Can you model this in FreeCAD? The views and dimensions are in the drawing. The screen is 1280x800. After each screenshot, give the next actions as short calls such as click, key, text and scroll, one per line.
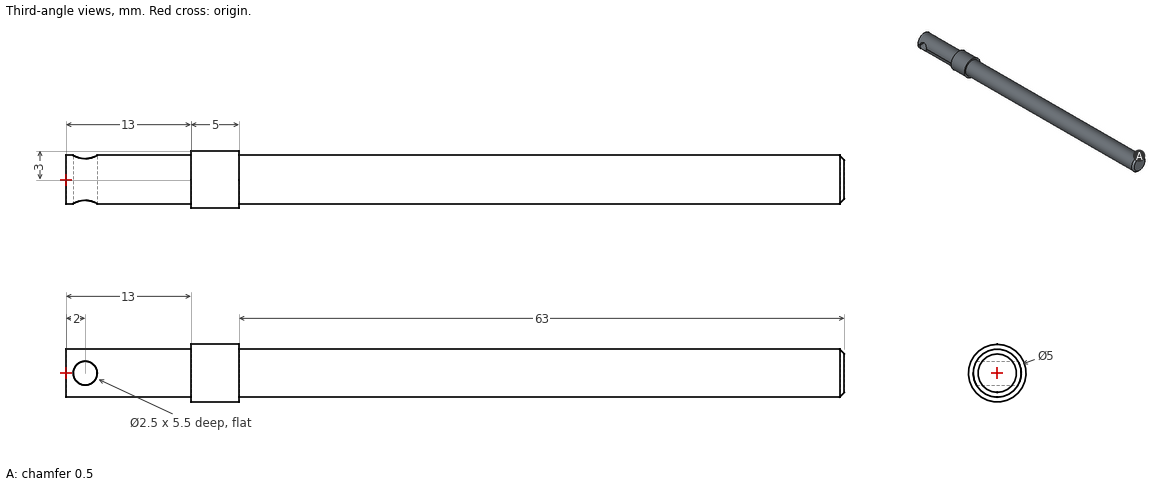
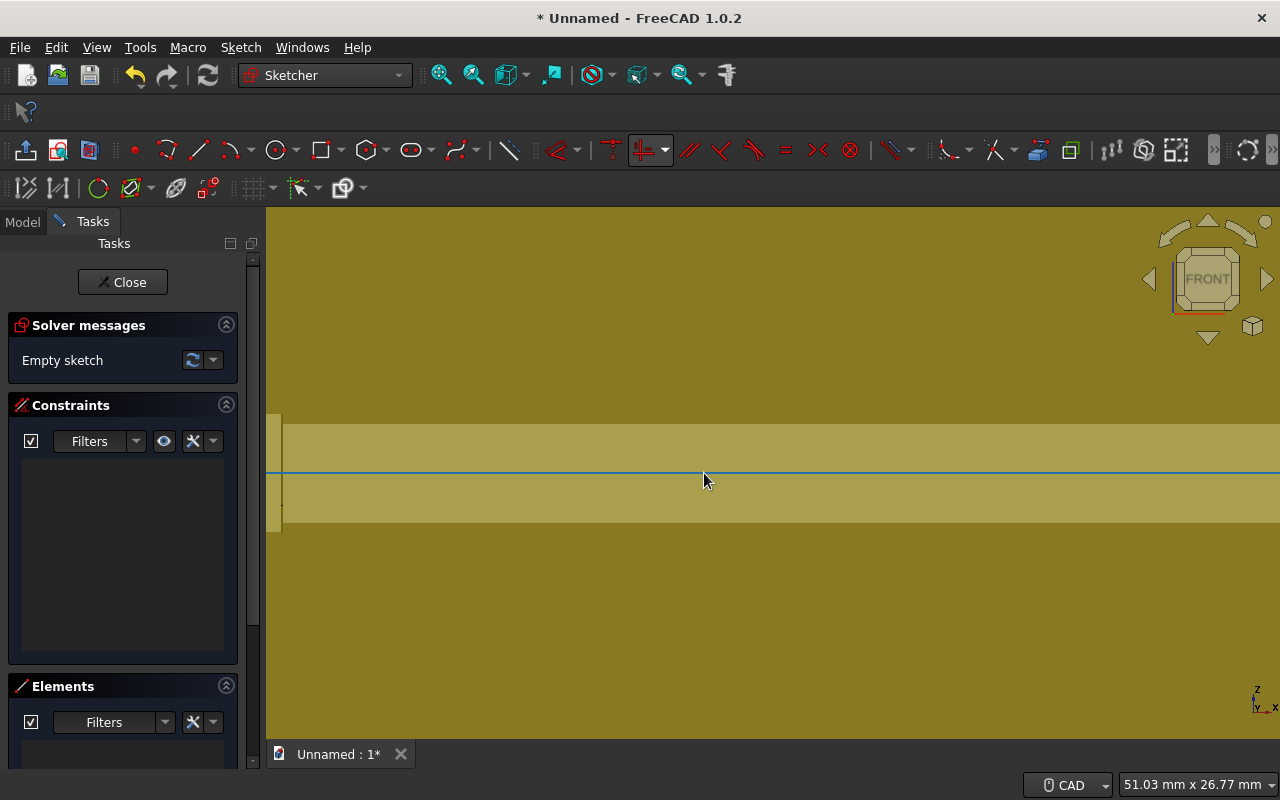
scroll(704, 473, down, 5)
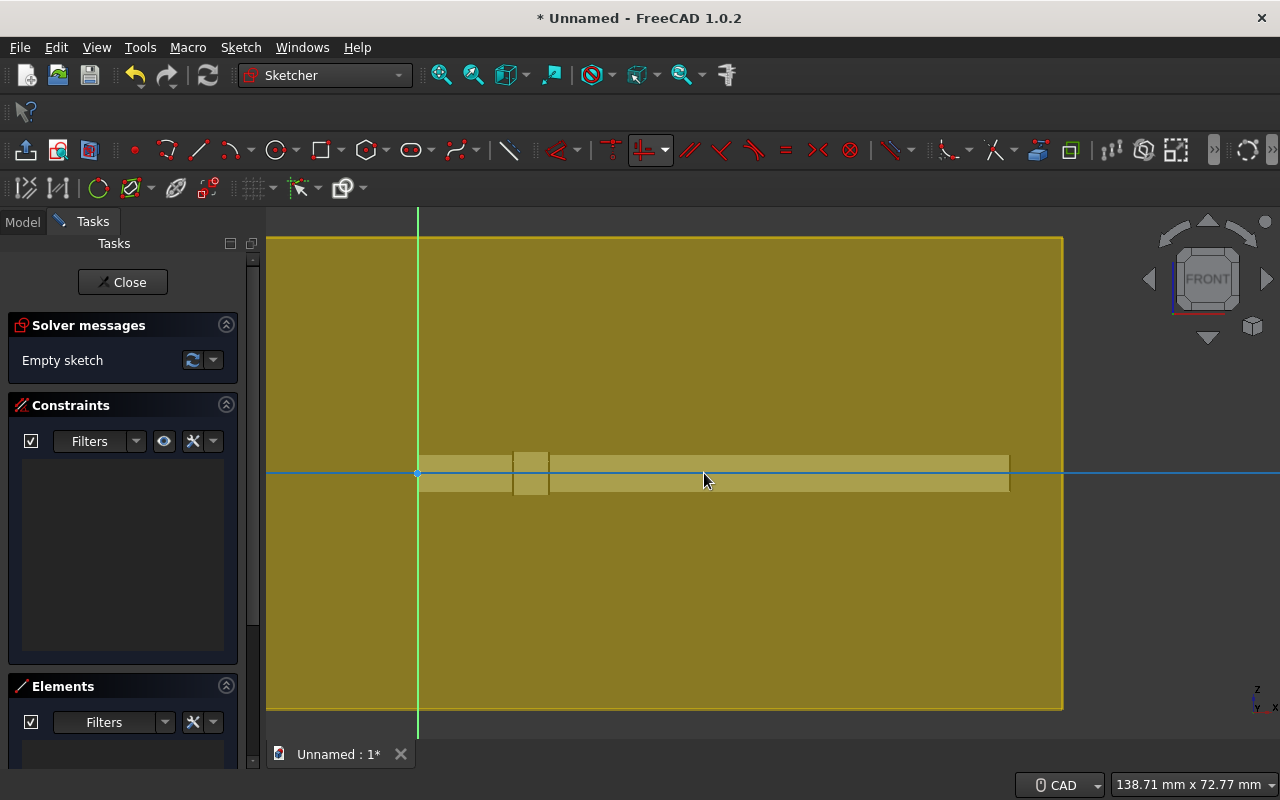
scroll(415, 473, up, 15)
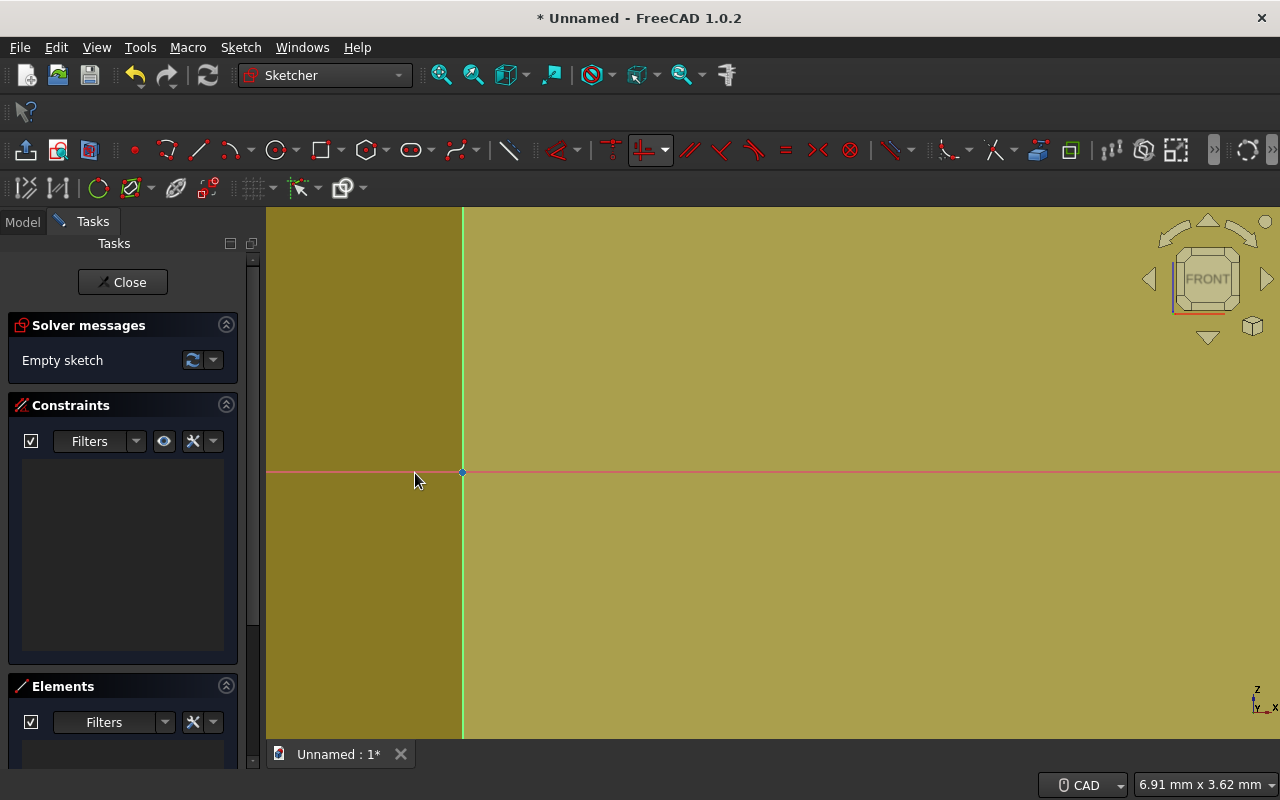
click(276, 150)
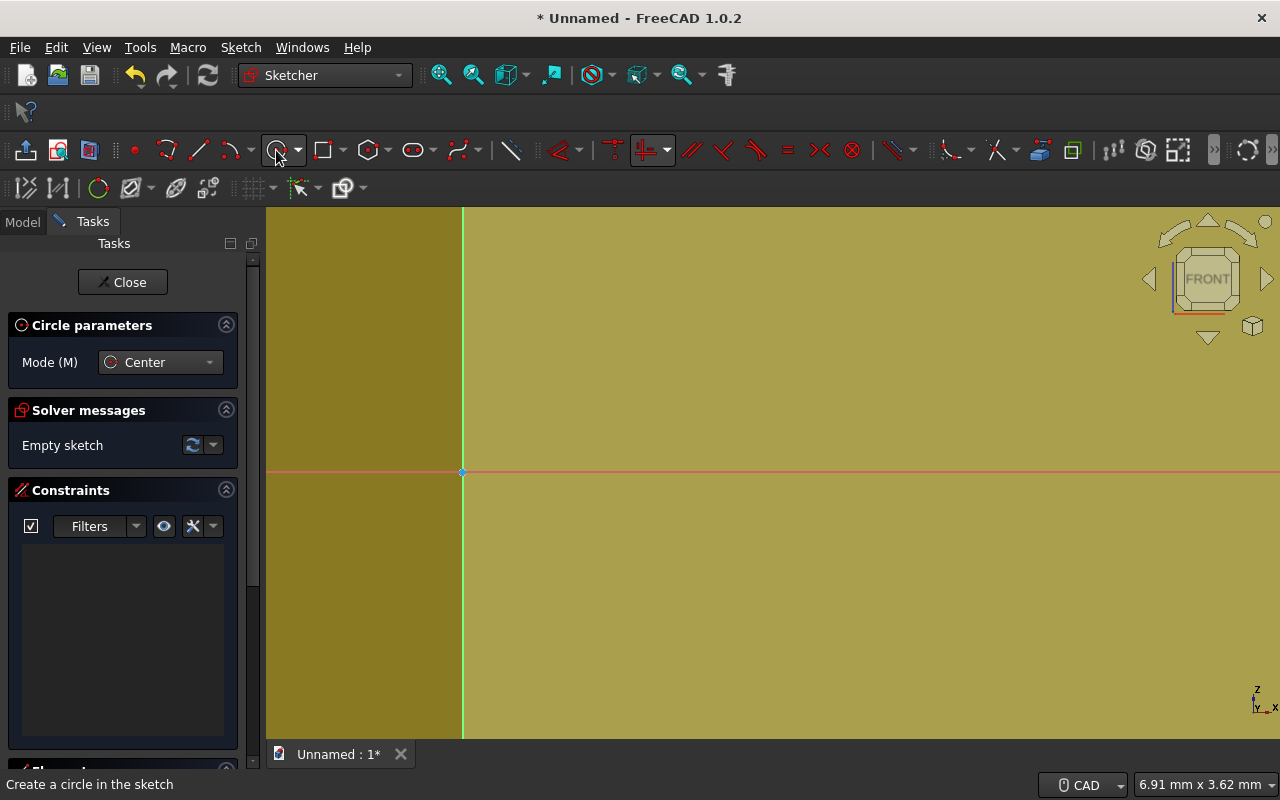
click(757, 472)
move(886, 342)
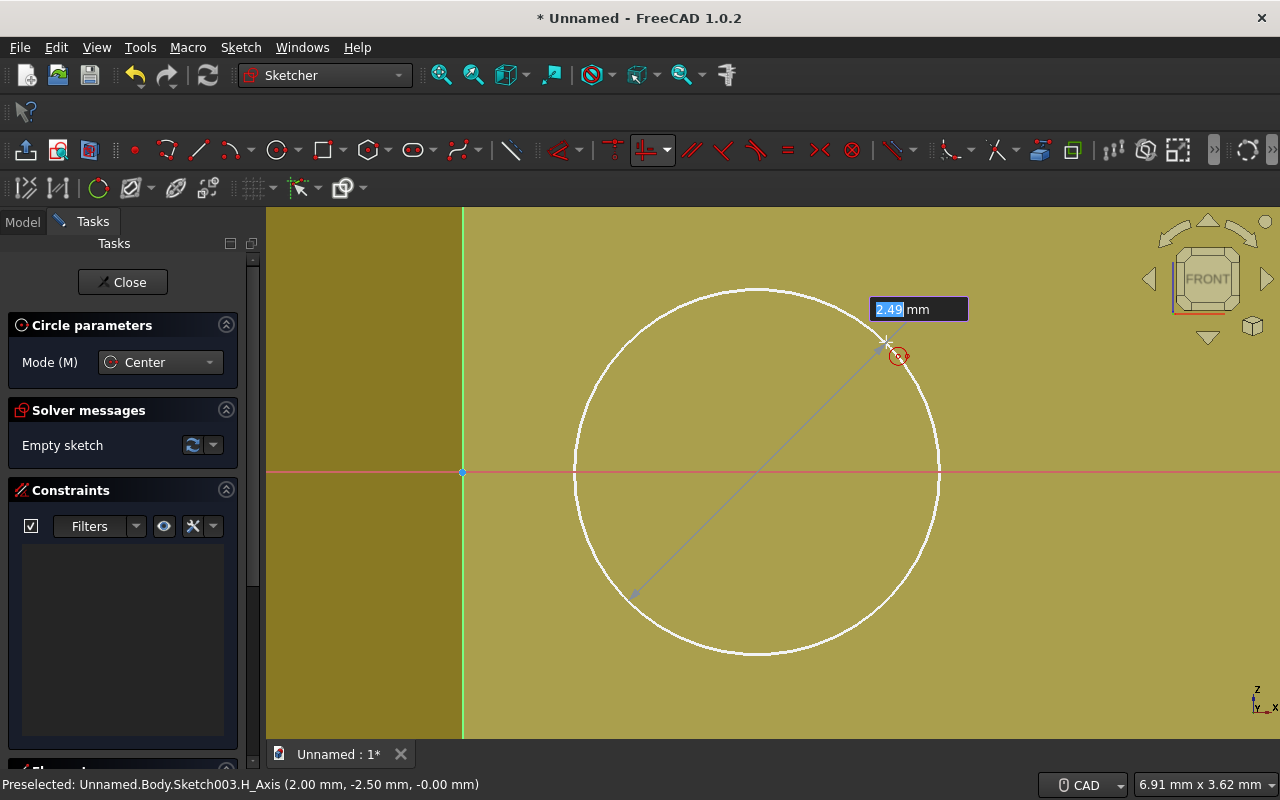
text(2.5)
key(Return)
key(Escape)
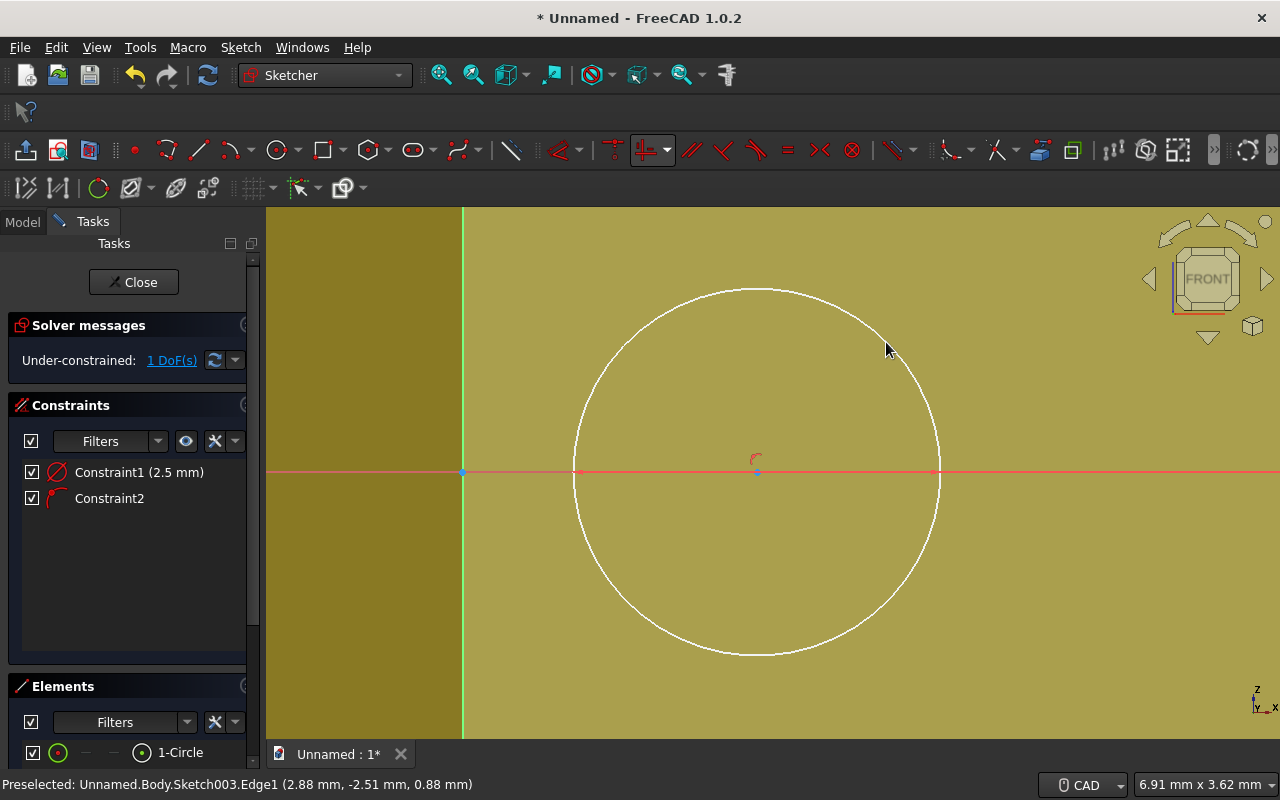
click(558, 150)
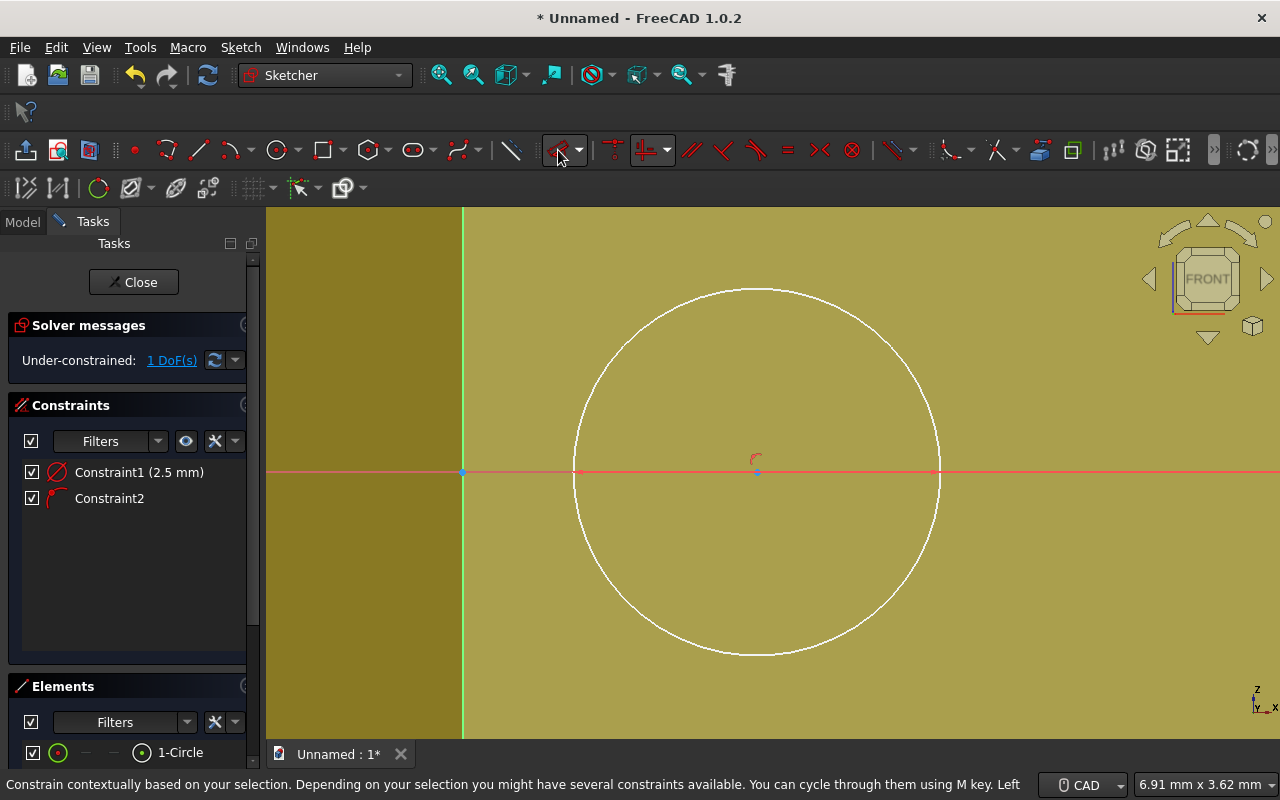
click(757, 472)
click(610, 506)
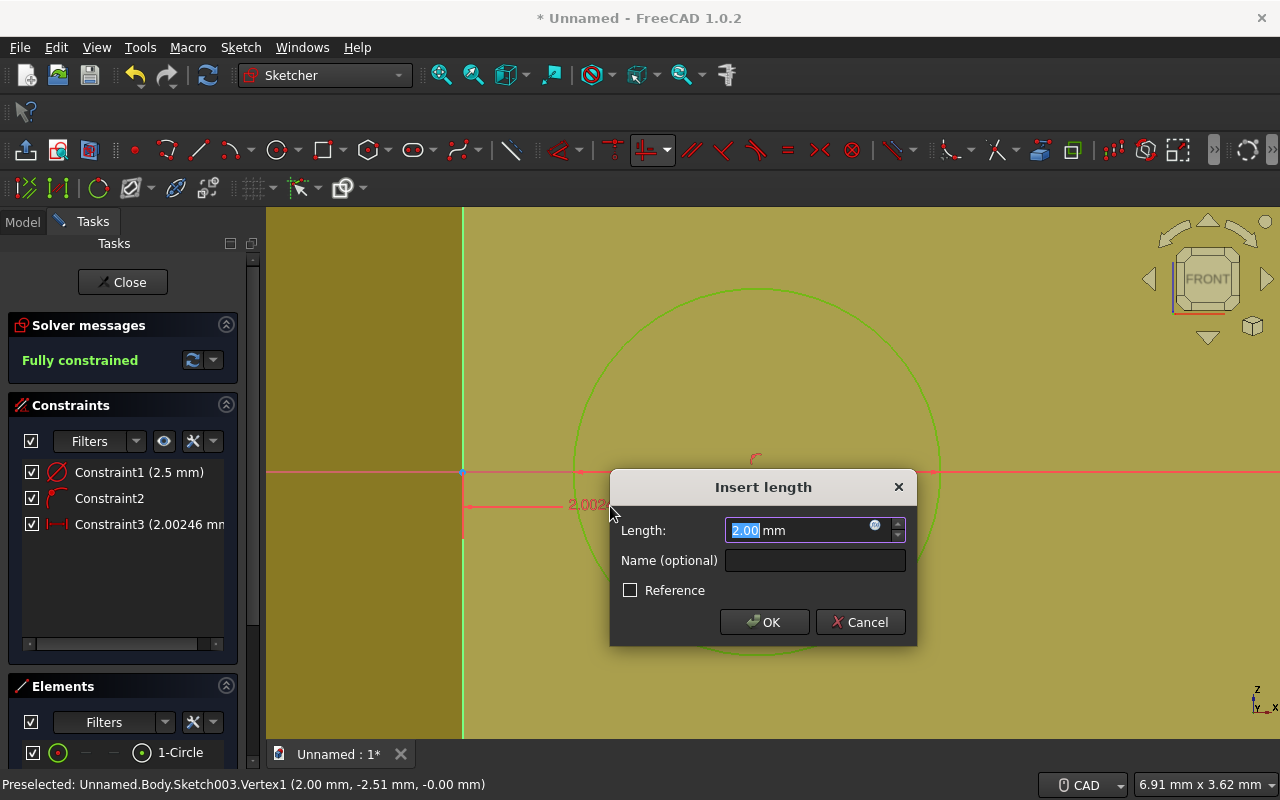
text(2)
key(Return)
key(Escape)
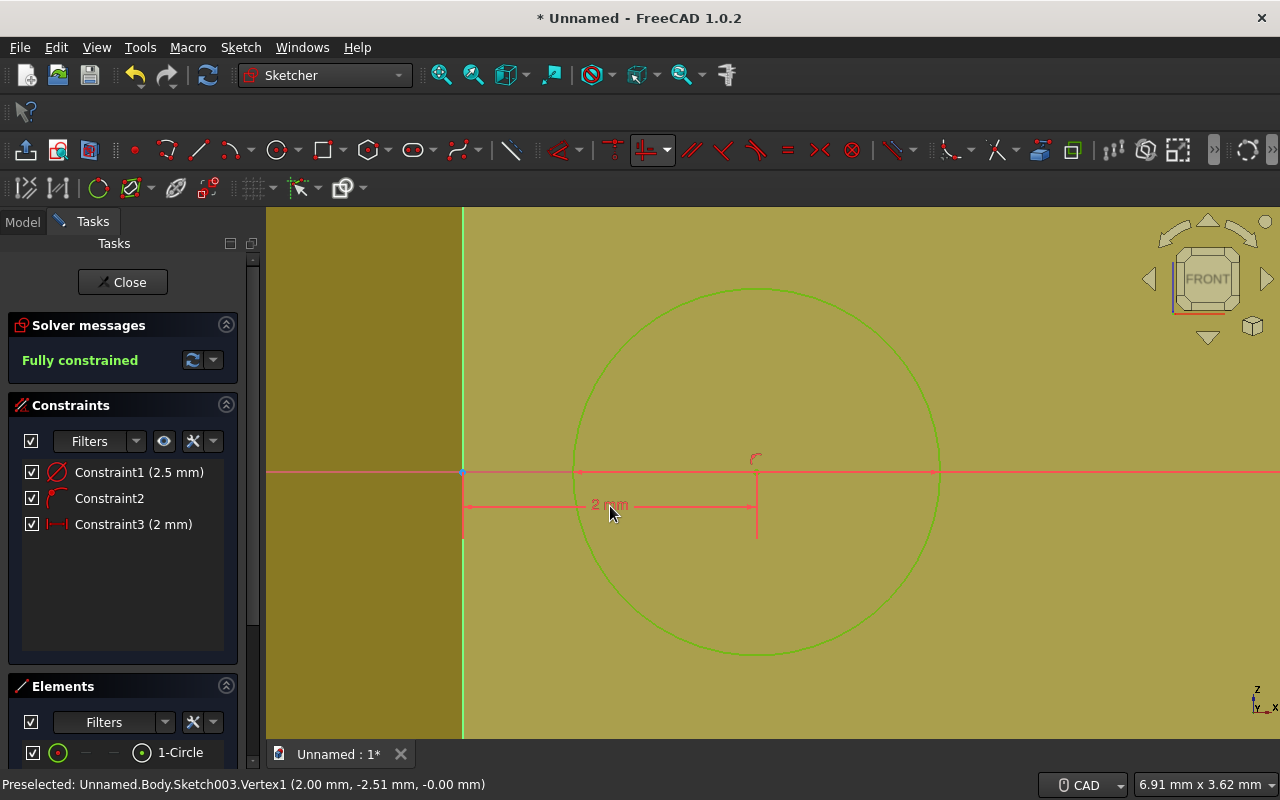
click(123, 282)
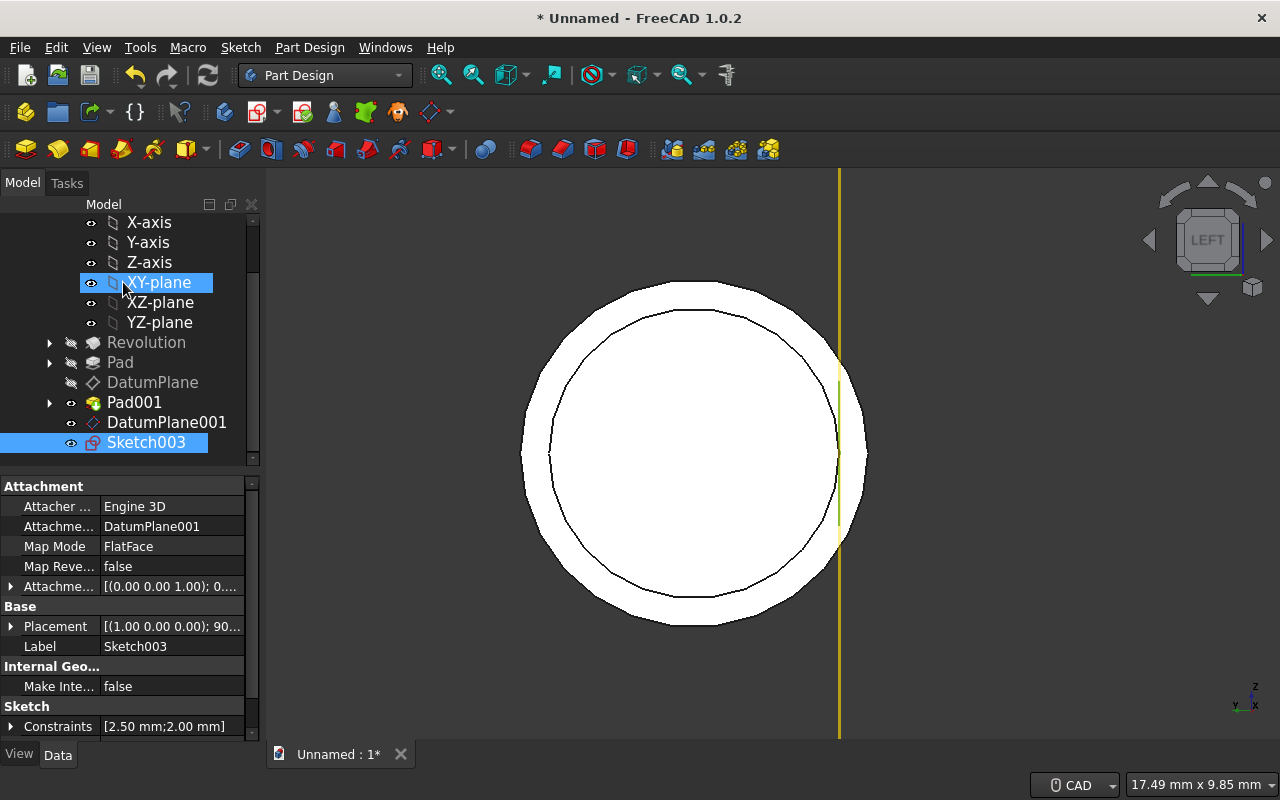
click(272, 150)